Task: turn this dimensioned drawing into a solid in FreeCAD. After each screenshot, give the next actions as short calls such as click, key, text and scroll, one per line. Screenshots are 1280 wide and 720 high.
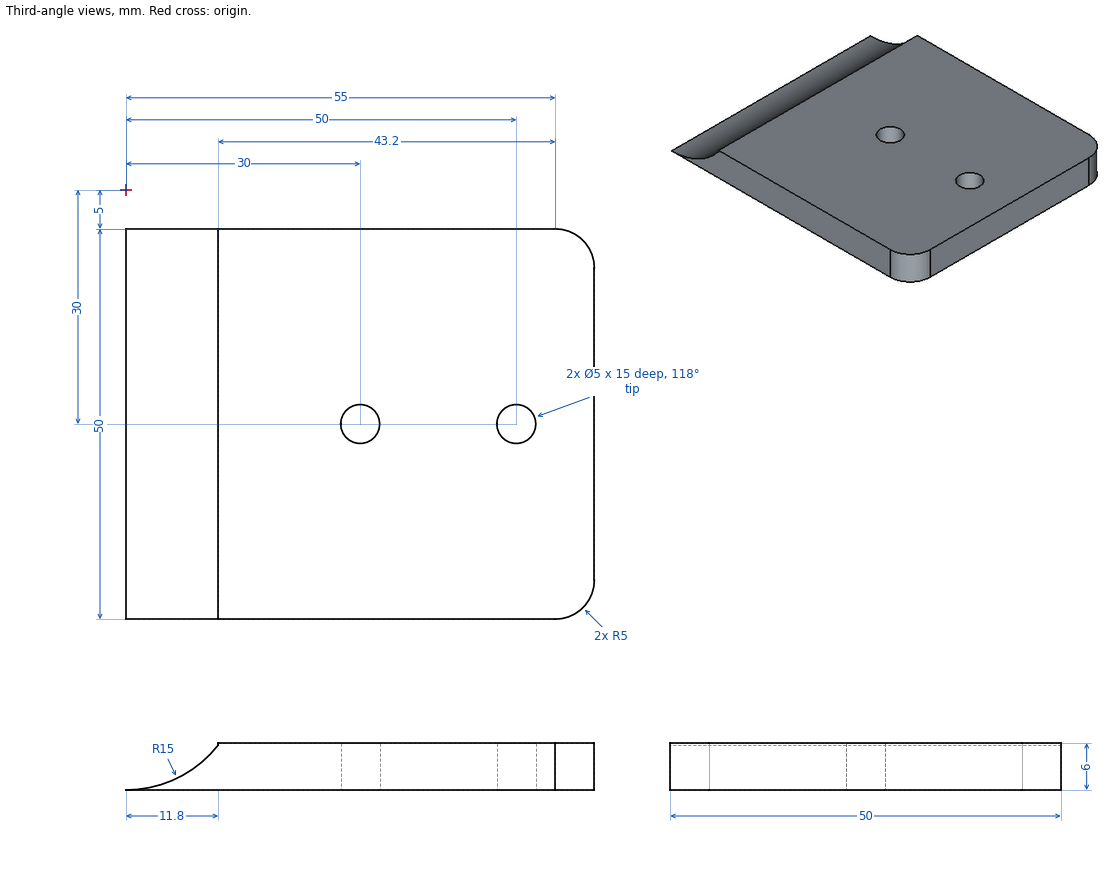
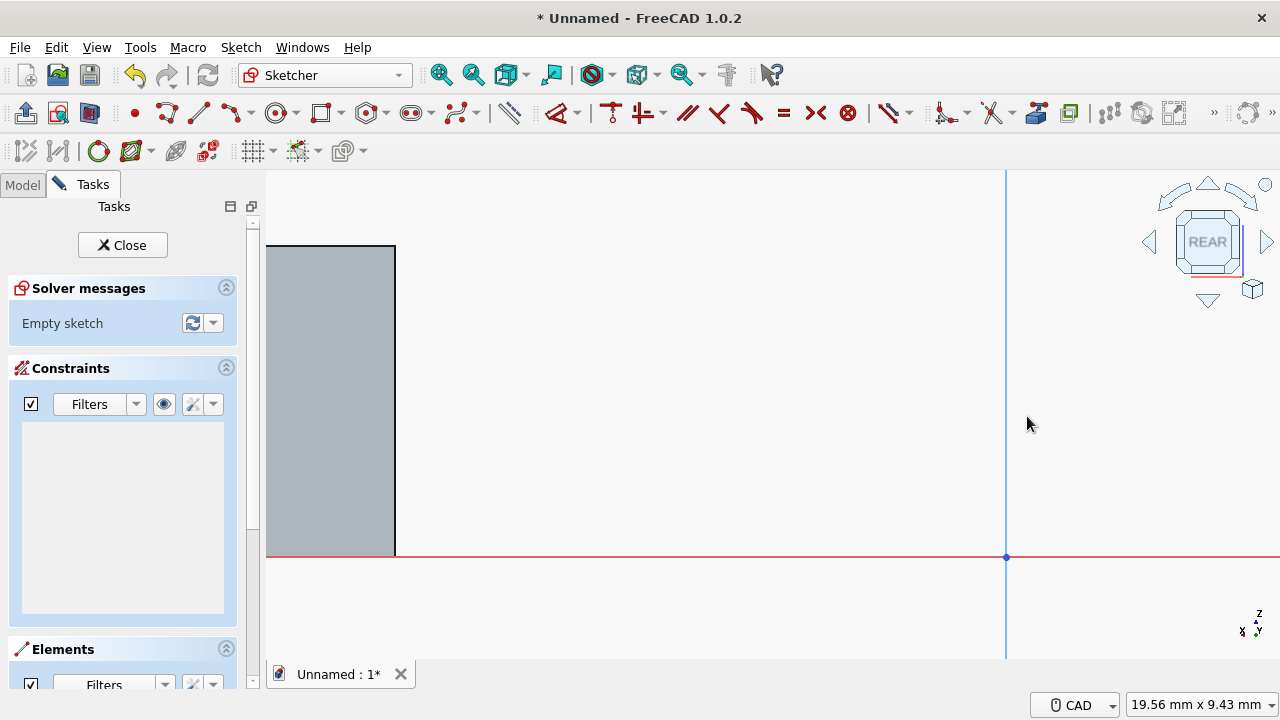
click(168, 114)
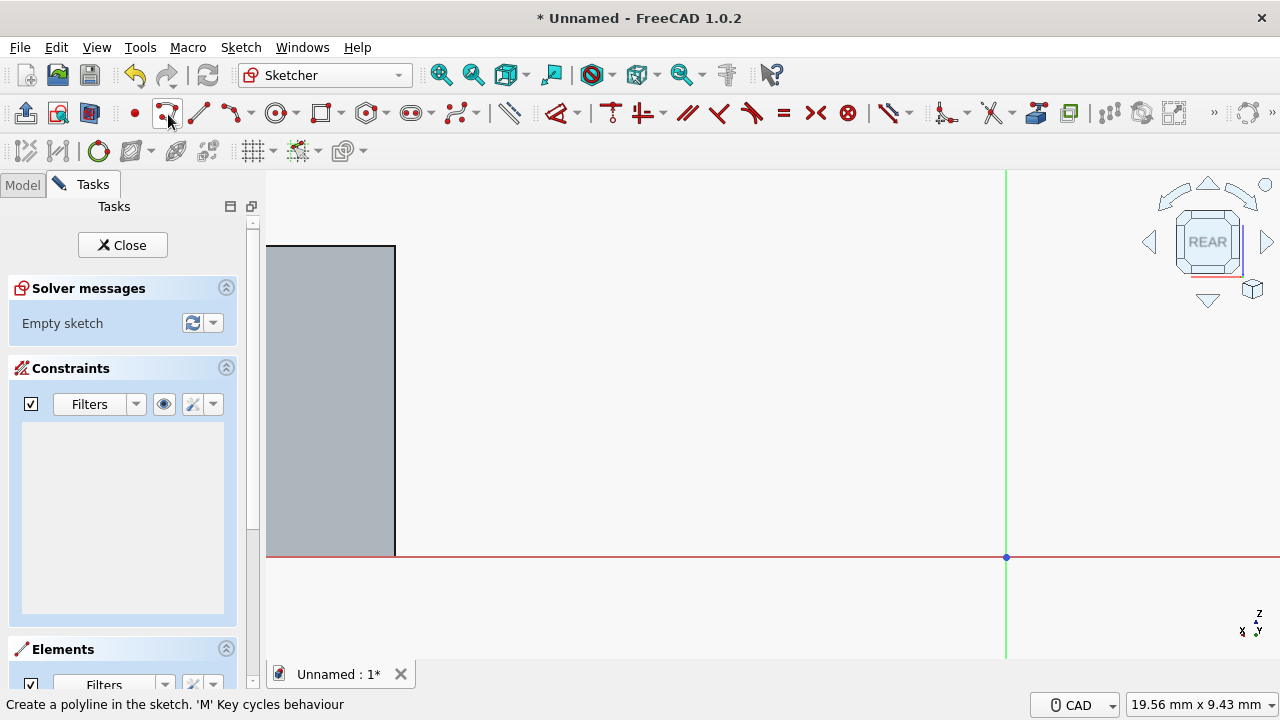
click(395, 260)
click(395, 557)
click(1006, 557)
right_click(1006, 557)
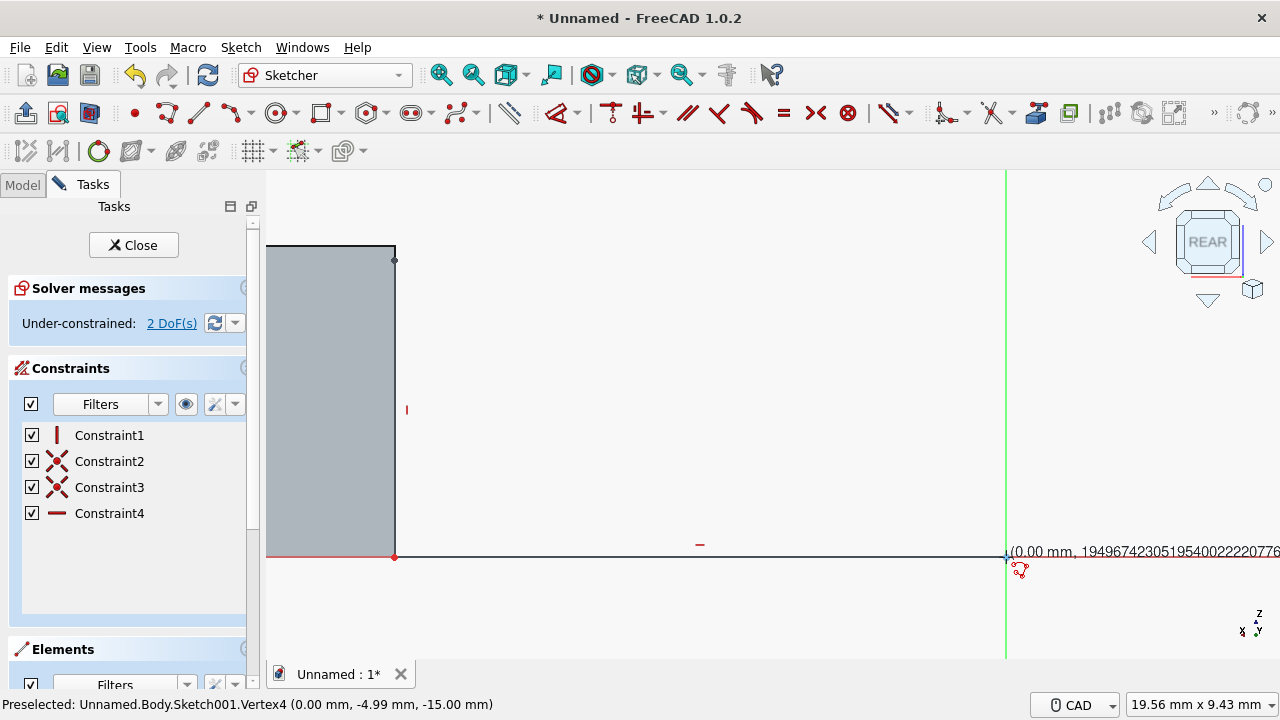
click(232, 114)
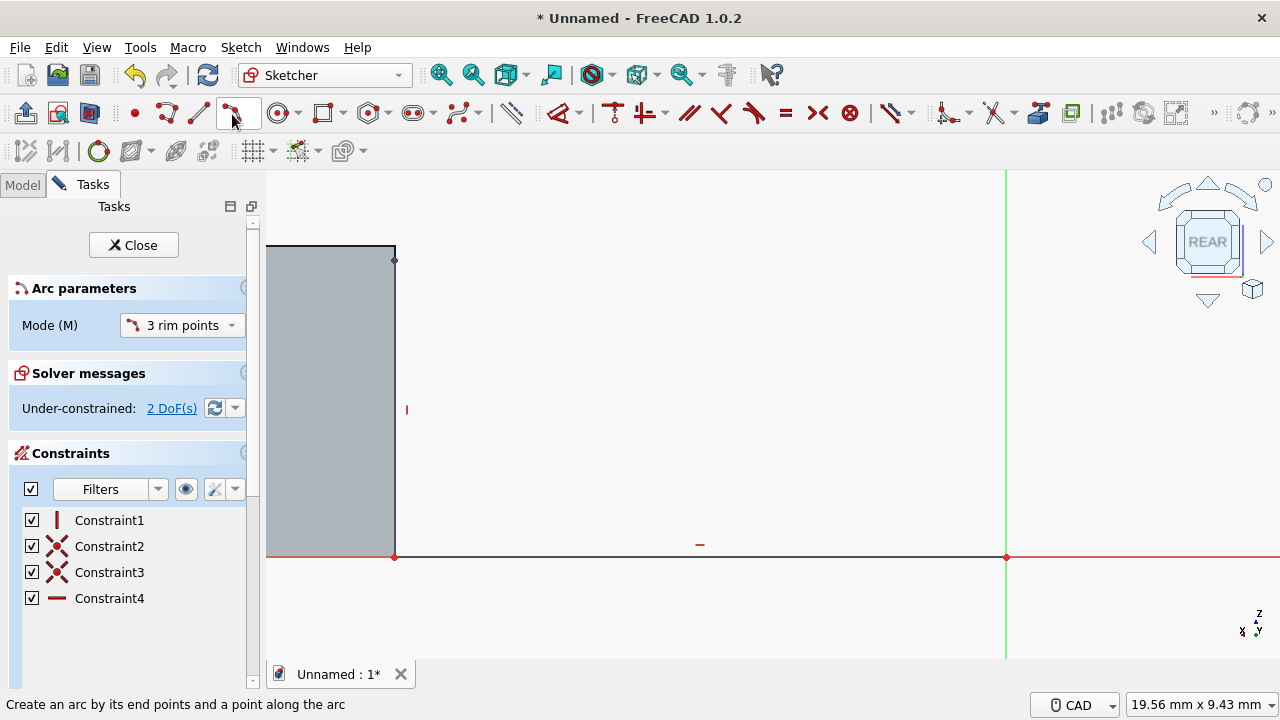
click(1006, 557)
click(395, 261)
click(666, 479)
key(Escape)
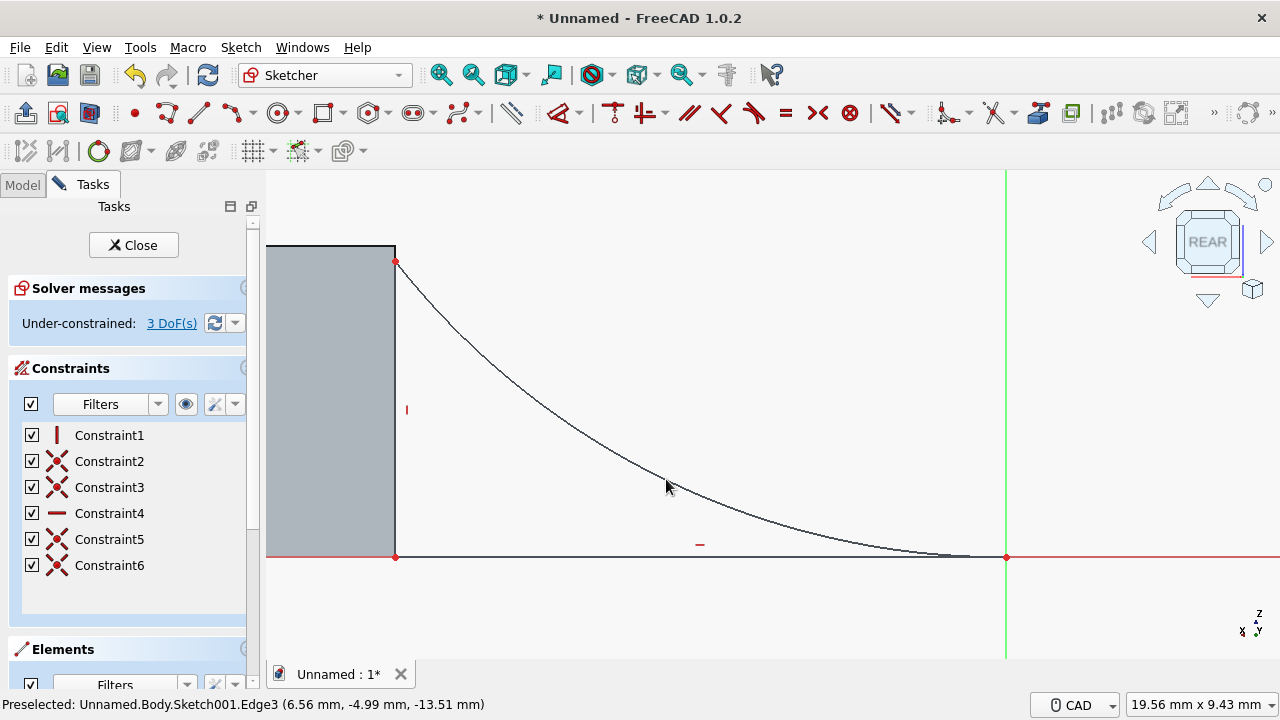
click(578, 557)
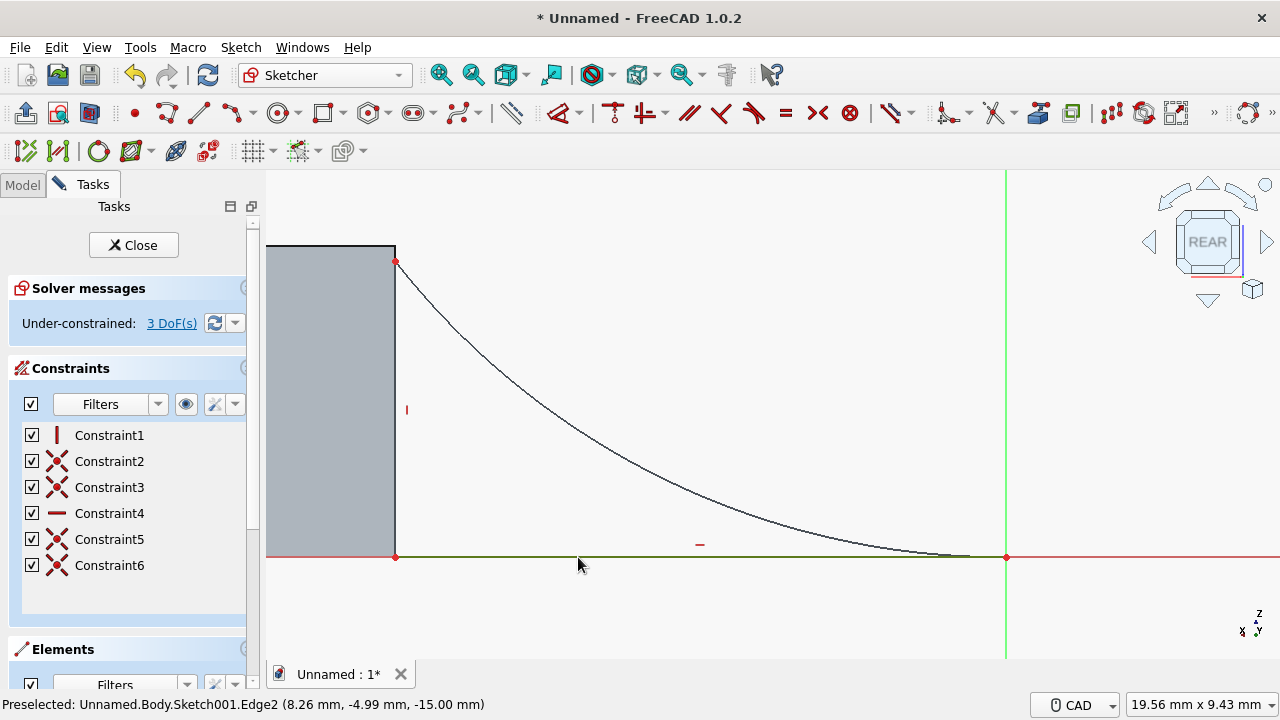
click(546, 408)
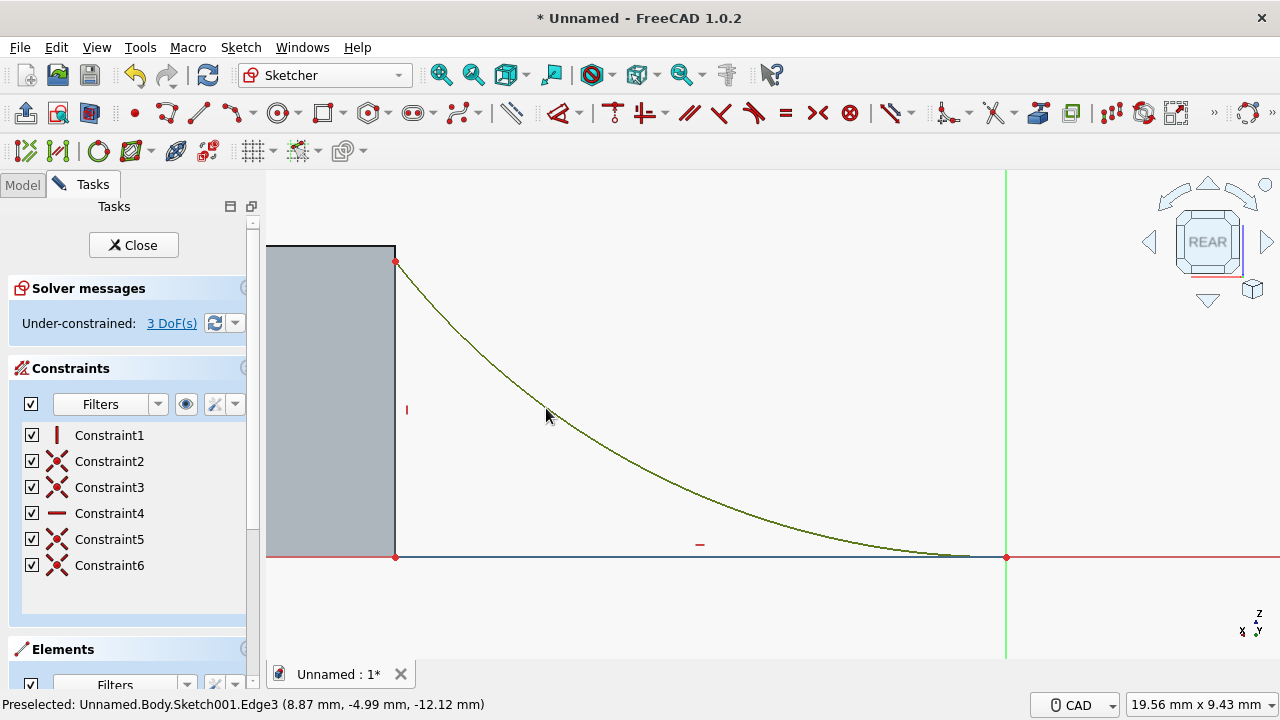
click(754, 114)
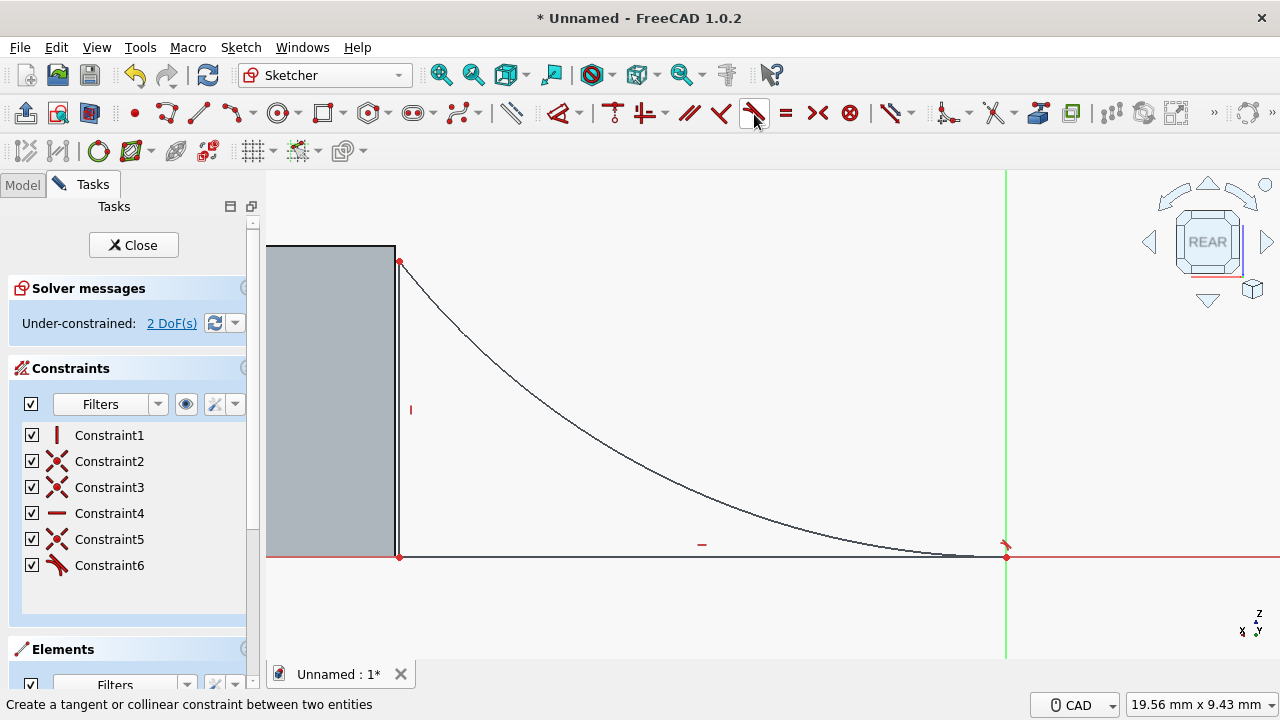
click(558, 114)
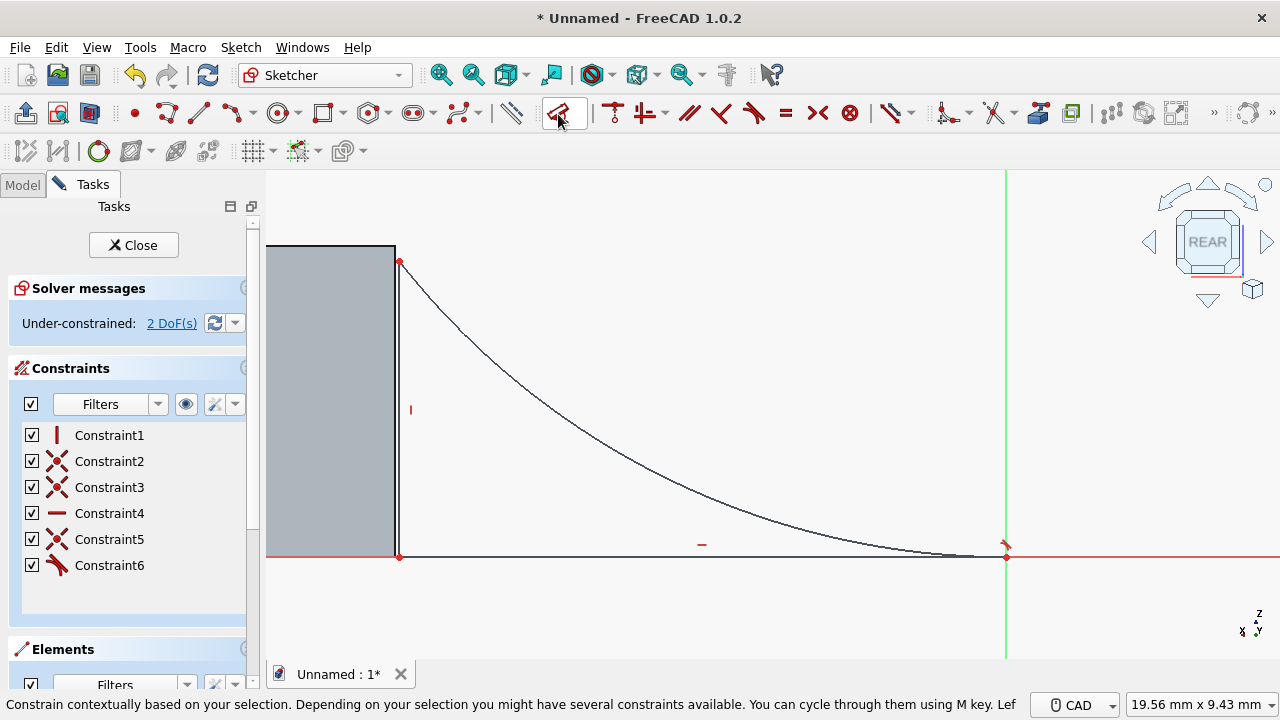
click(549, 407)
click(530, 433)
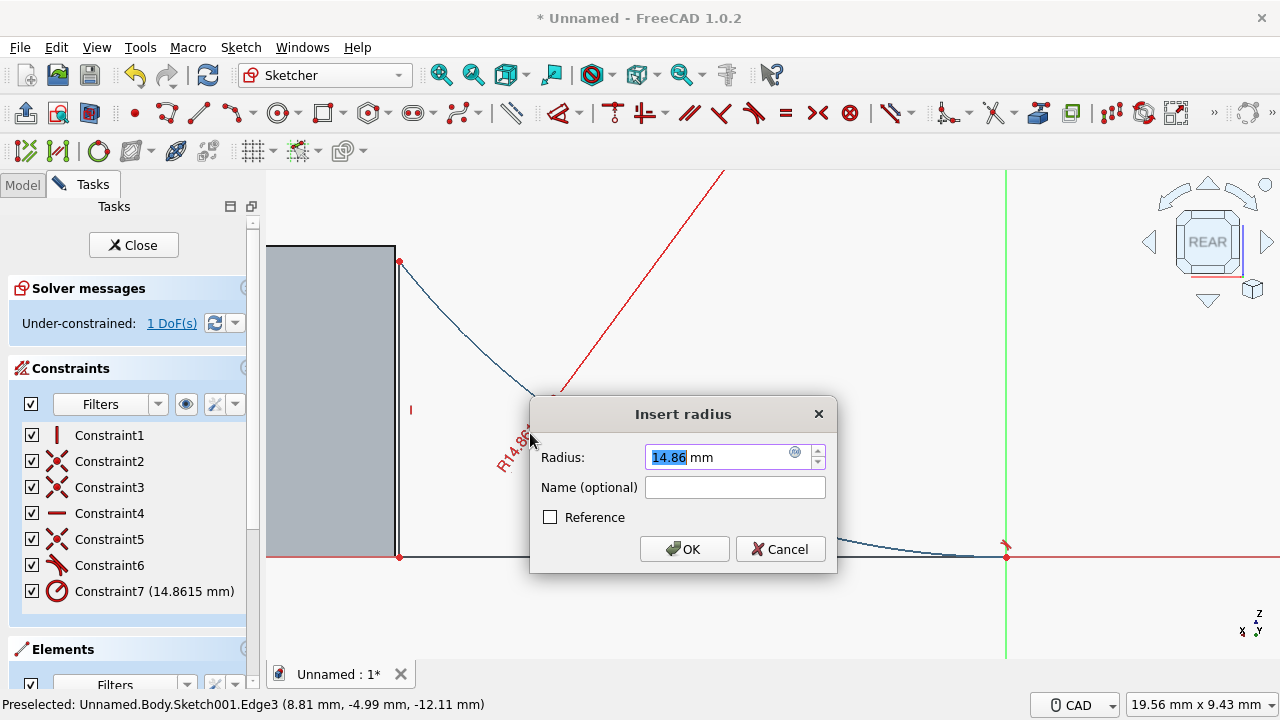
text(15)
key(Return)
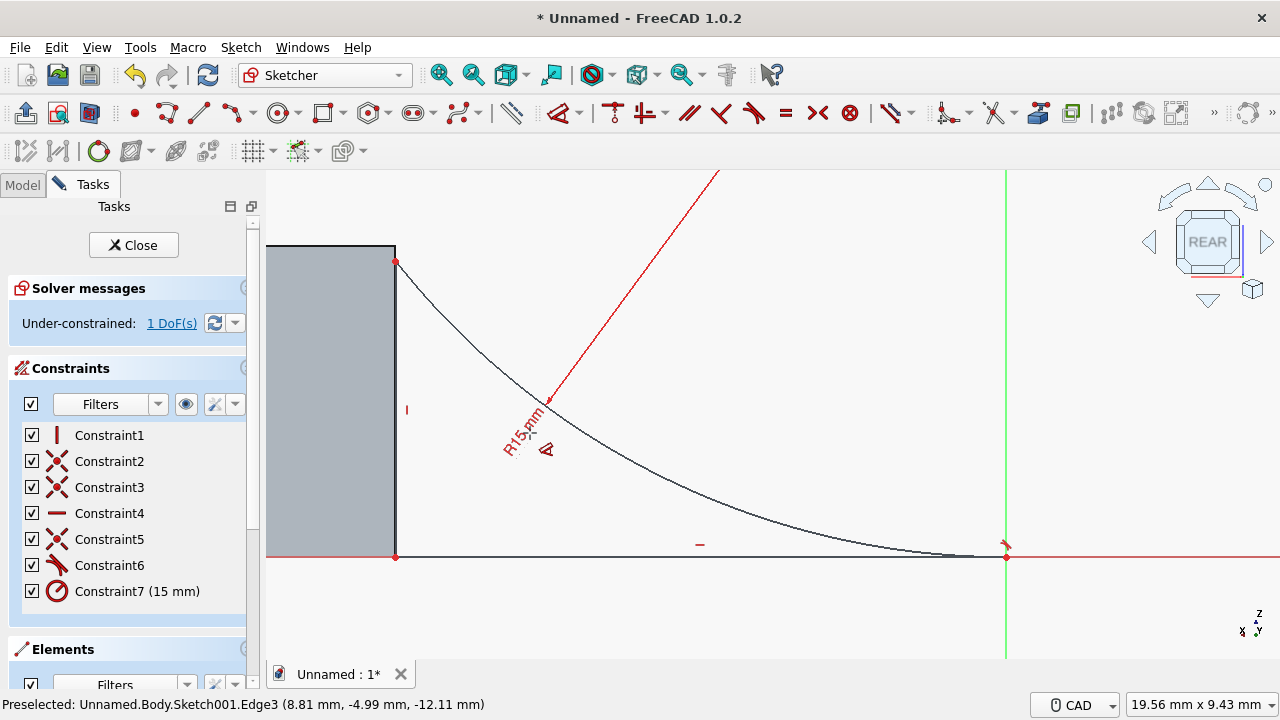
click(579, 557)
click(701, 591)